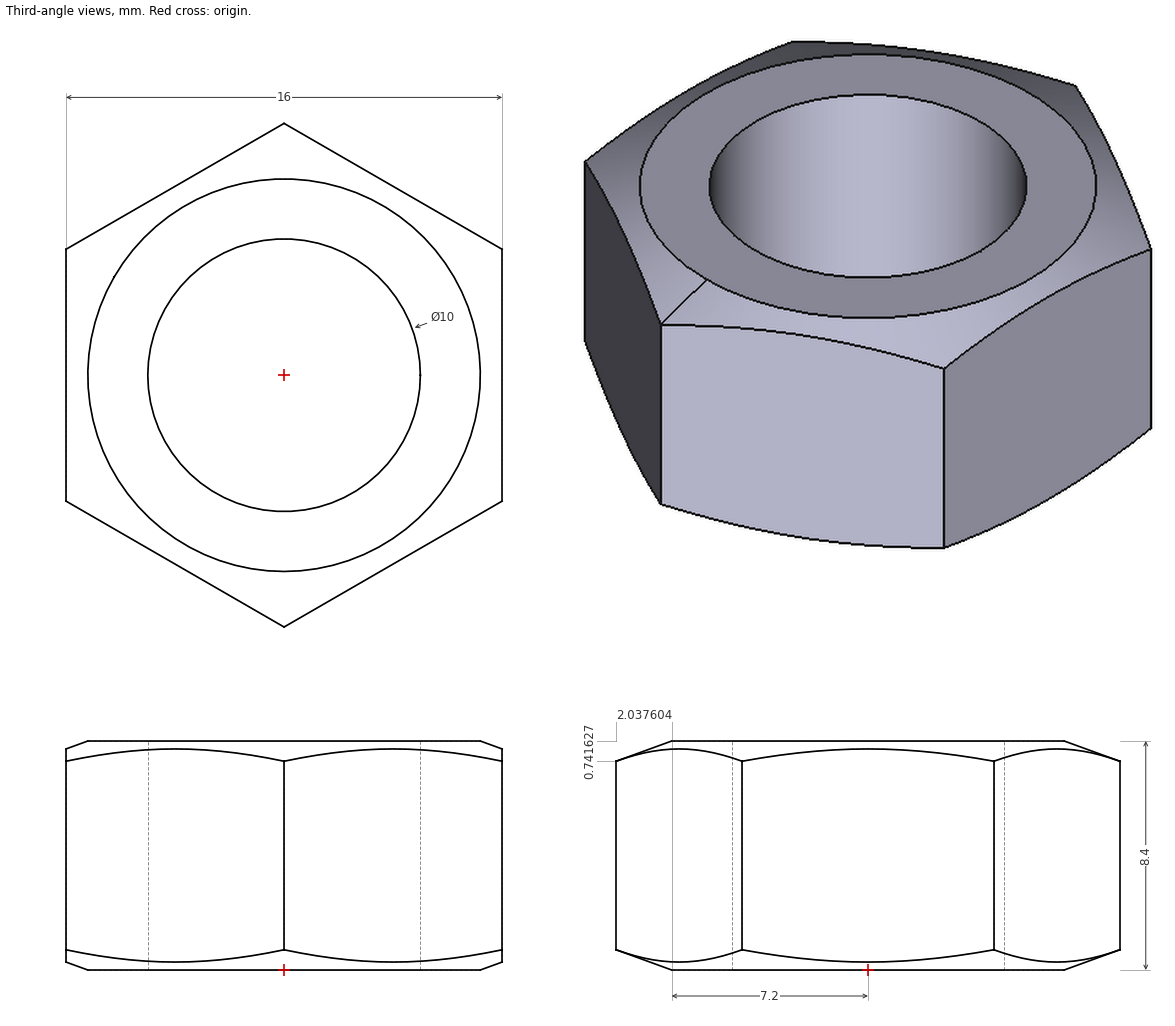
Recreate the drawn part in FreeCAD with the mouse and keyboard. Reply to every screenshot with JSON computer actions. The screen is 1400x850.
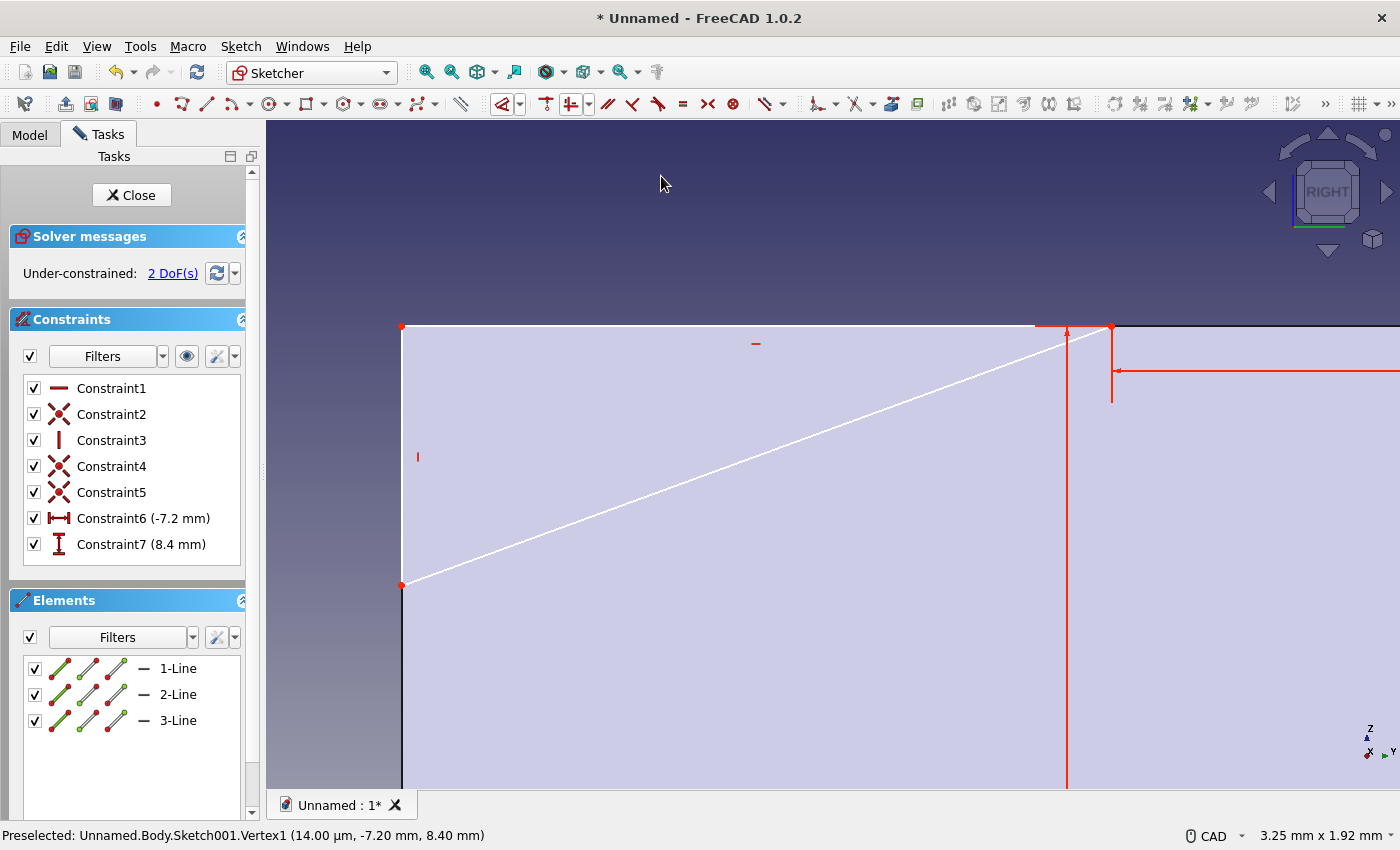
{"action": "left_click", "coordinate": [899, 326]}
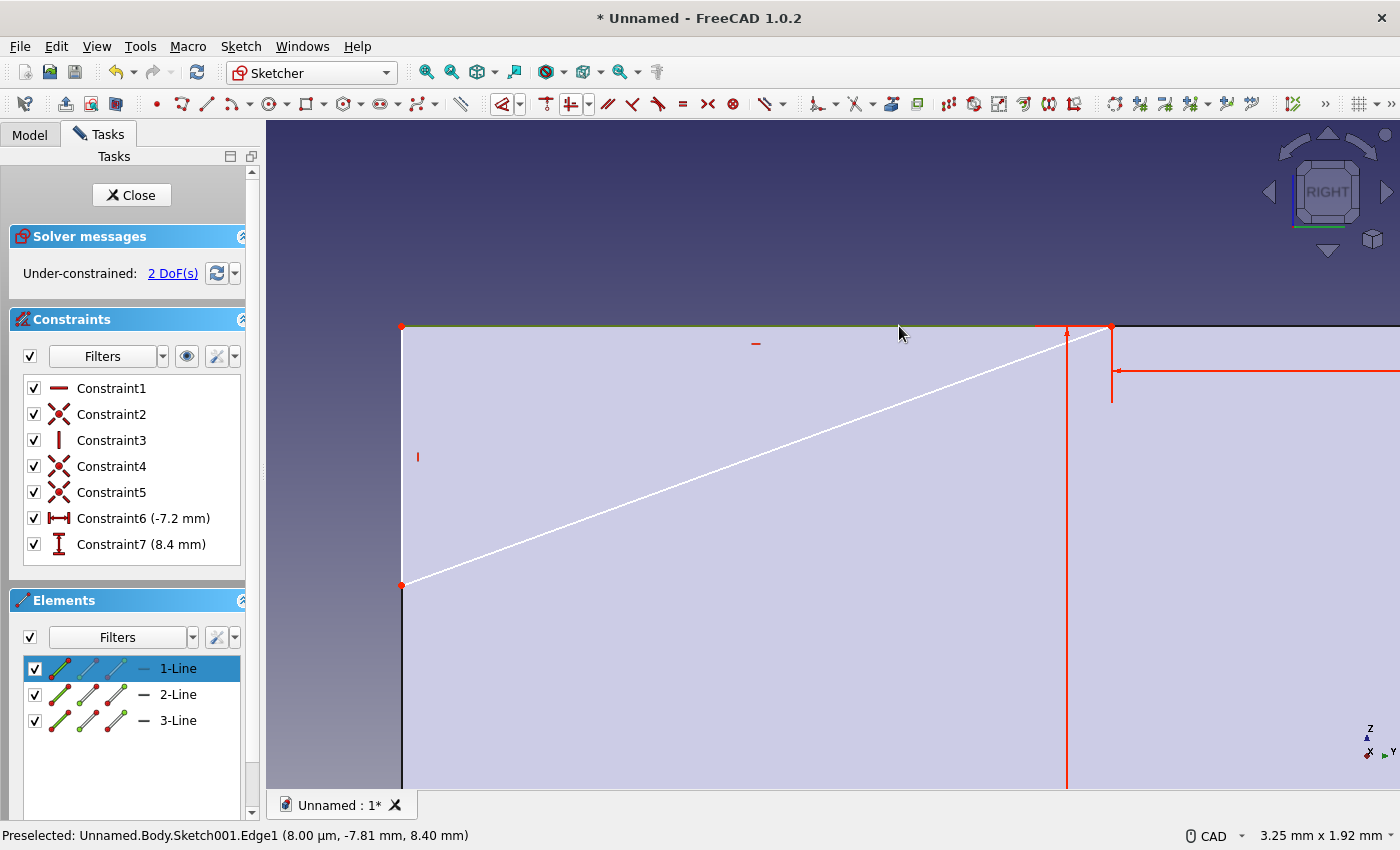
{"action": "key", "text": "l"}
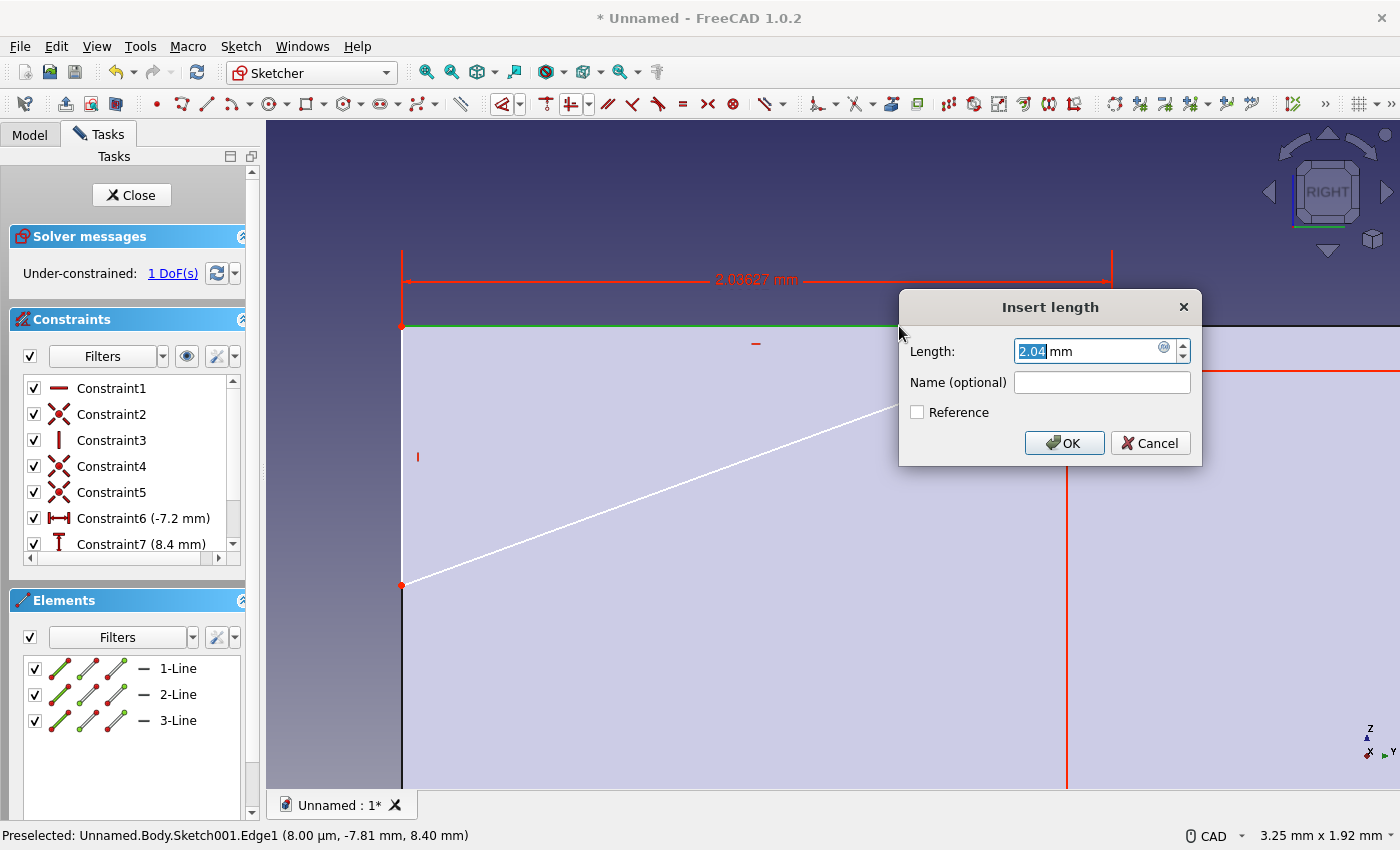
{"action": "type", "text": "2.037604"}
{"action": "key", "text": "Return"}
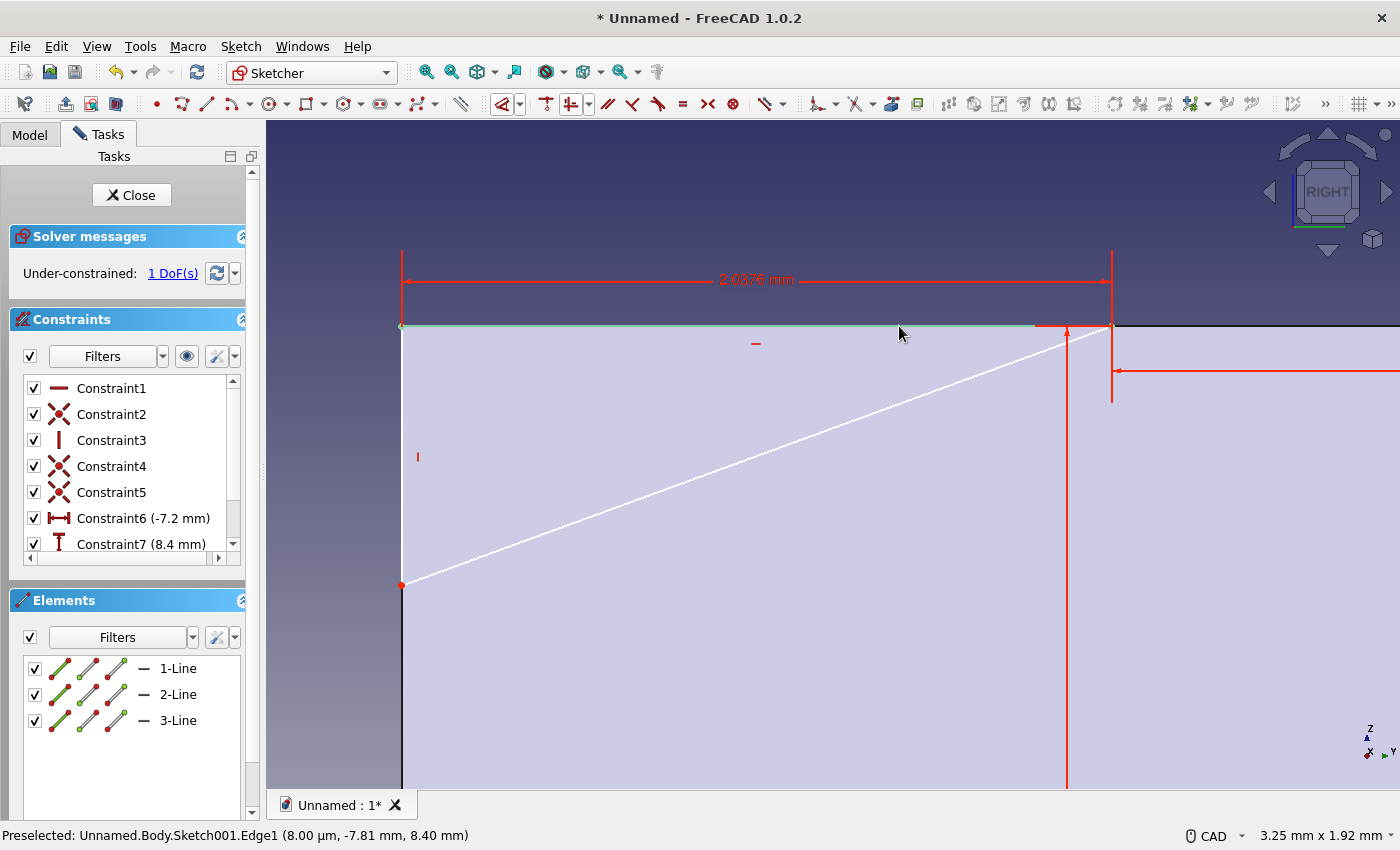
{"action": "left_click", "coordinate": [402, 404]}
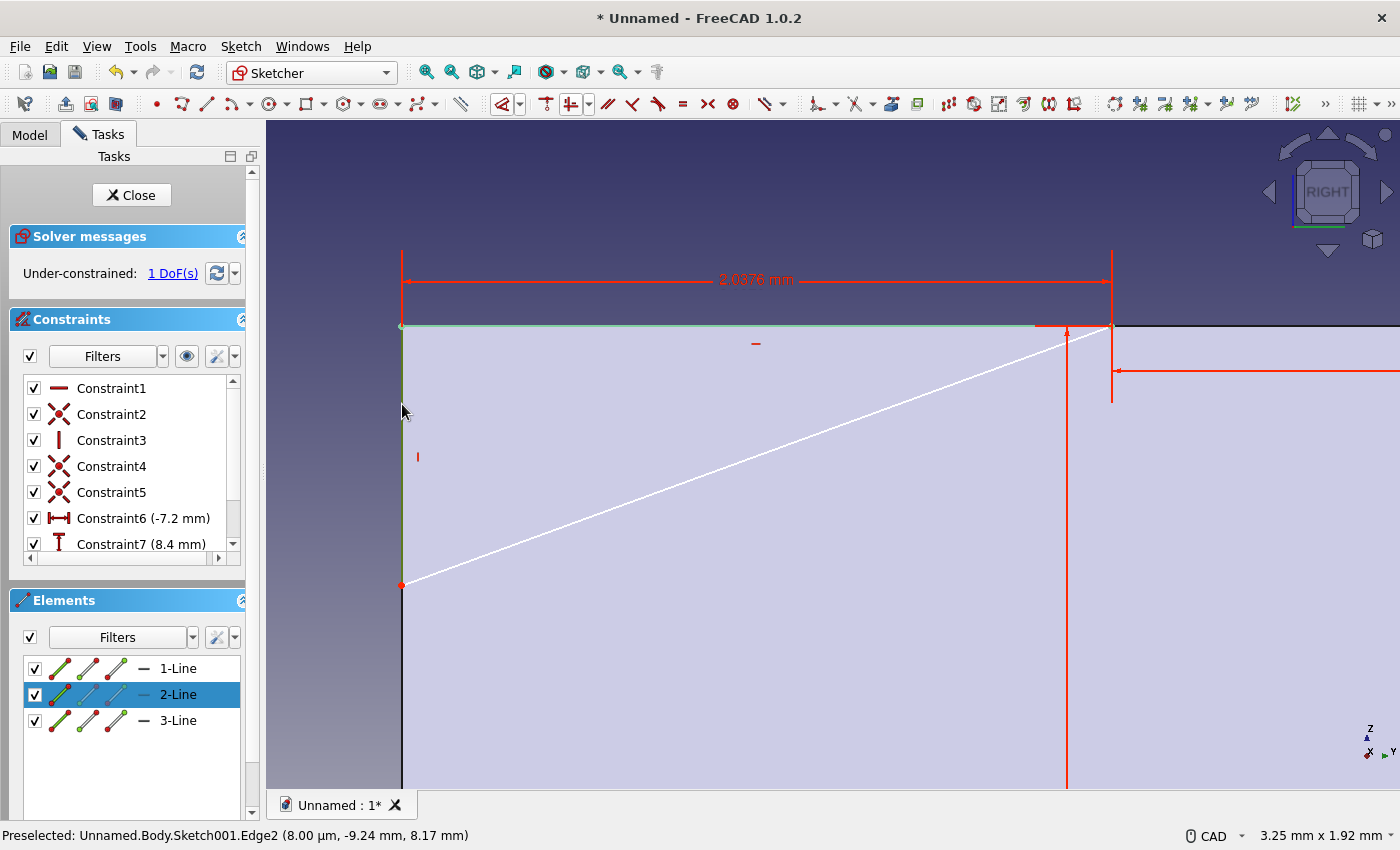
{"action": "key", "text": "i"}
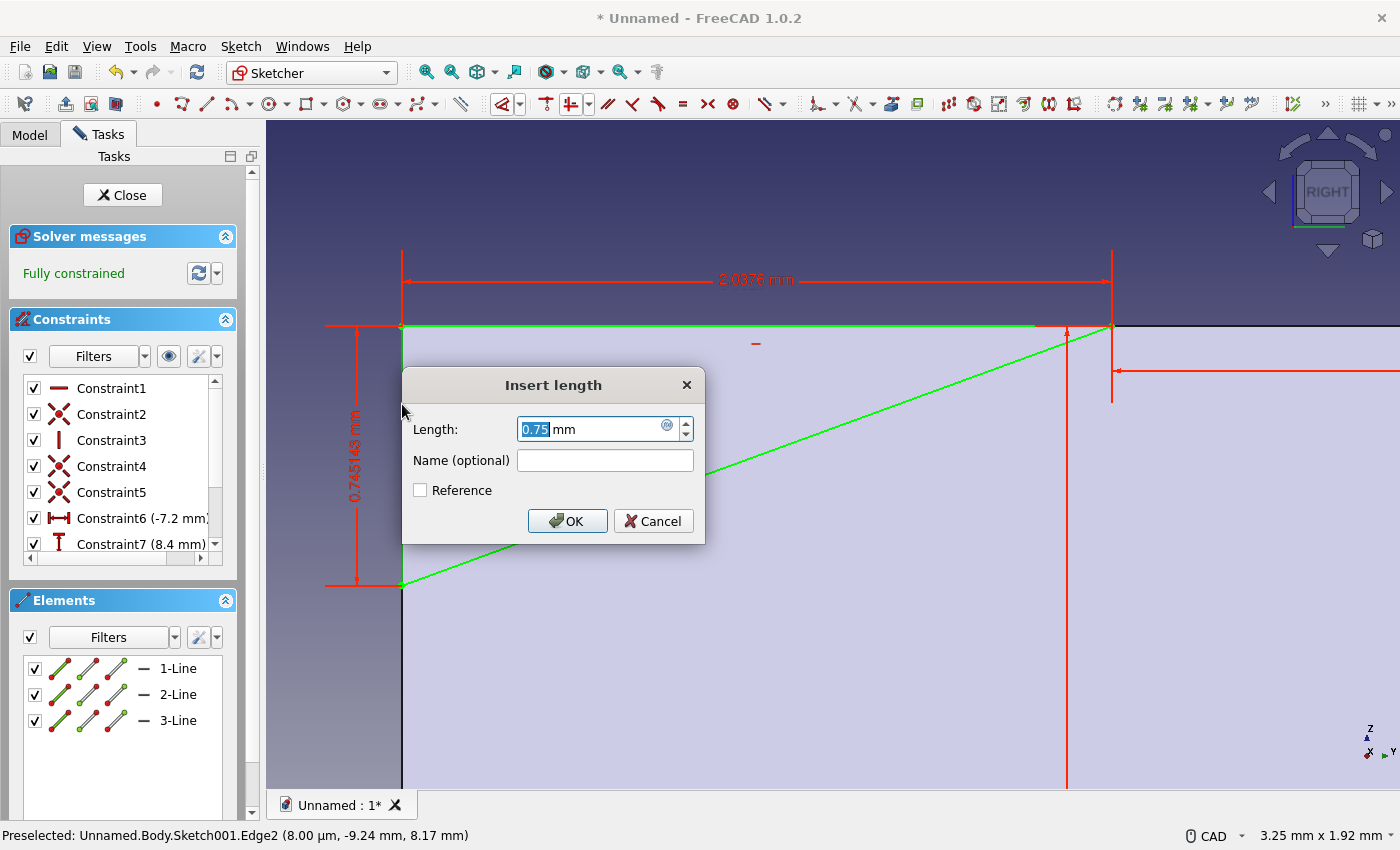
{"action": "type", "text": "0.741627"}
{"action": "key", "text": "Return"}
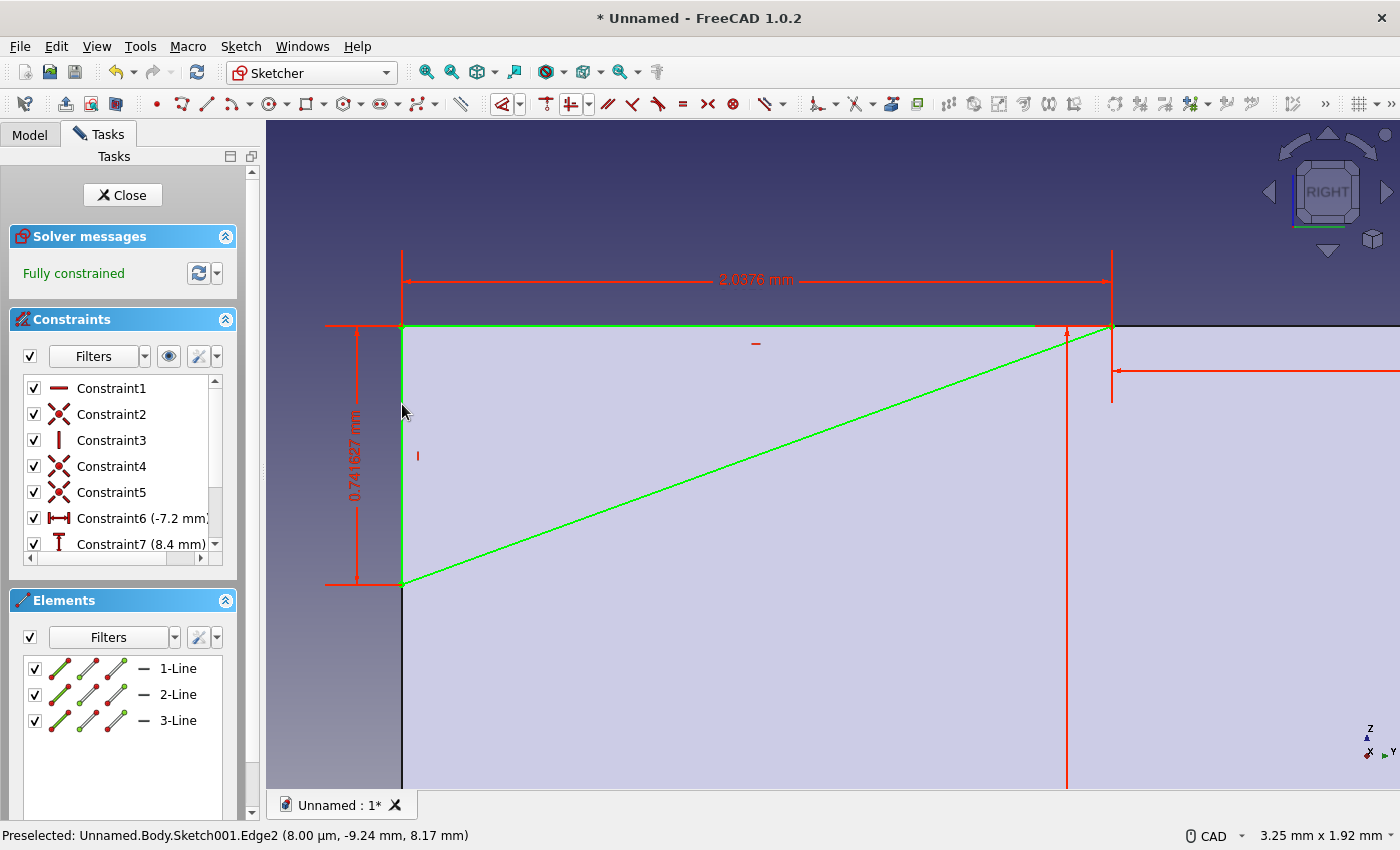
{"action": "left_click", "coordinate": [123, 195]}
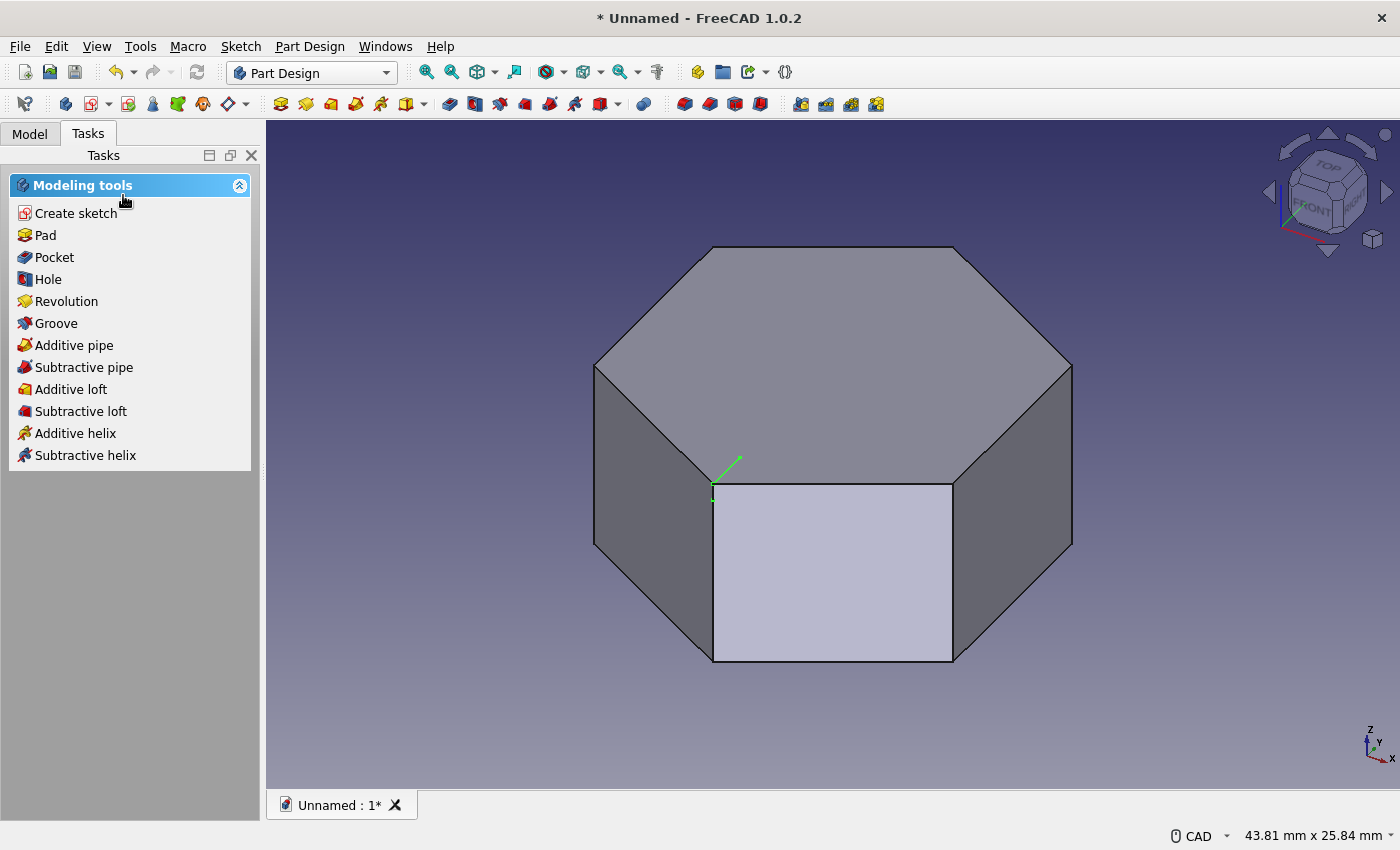
{"action": "left_click", "coordinate": [500, 104]}